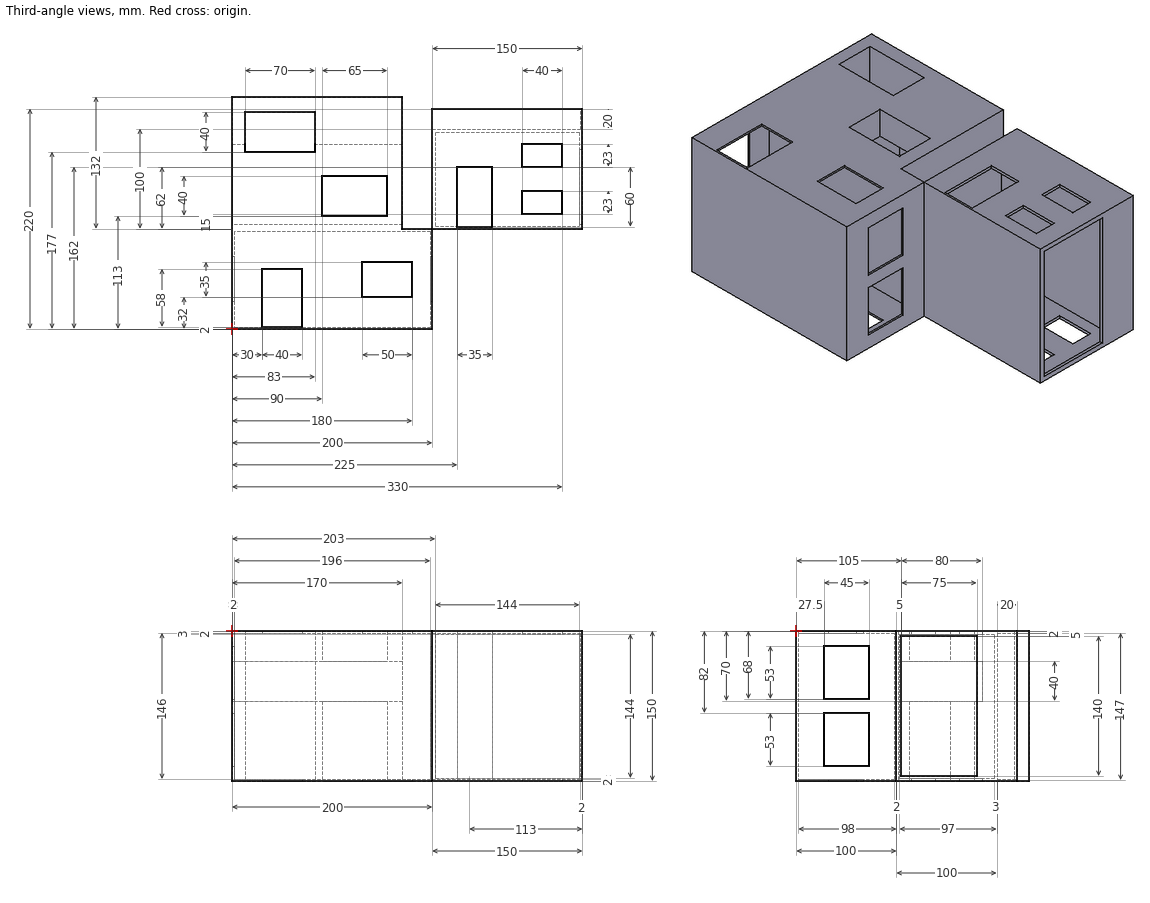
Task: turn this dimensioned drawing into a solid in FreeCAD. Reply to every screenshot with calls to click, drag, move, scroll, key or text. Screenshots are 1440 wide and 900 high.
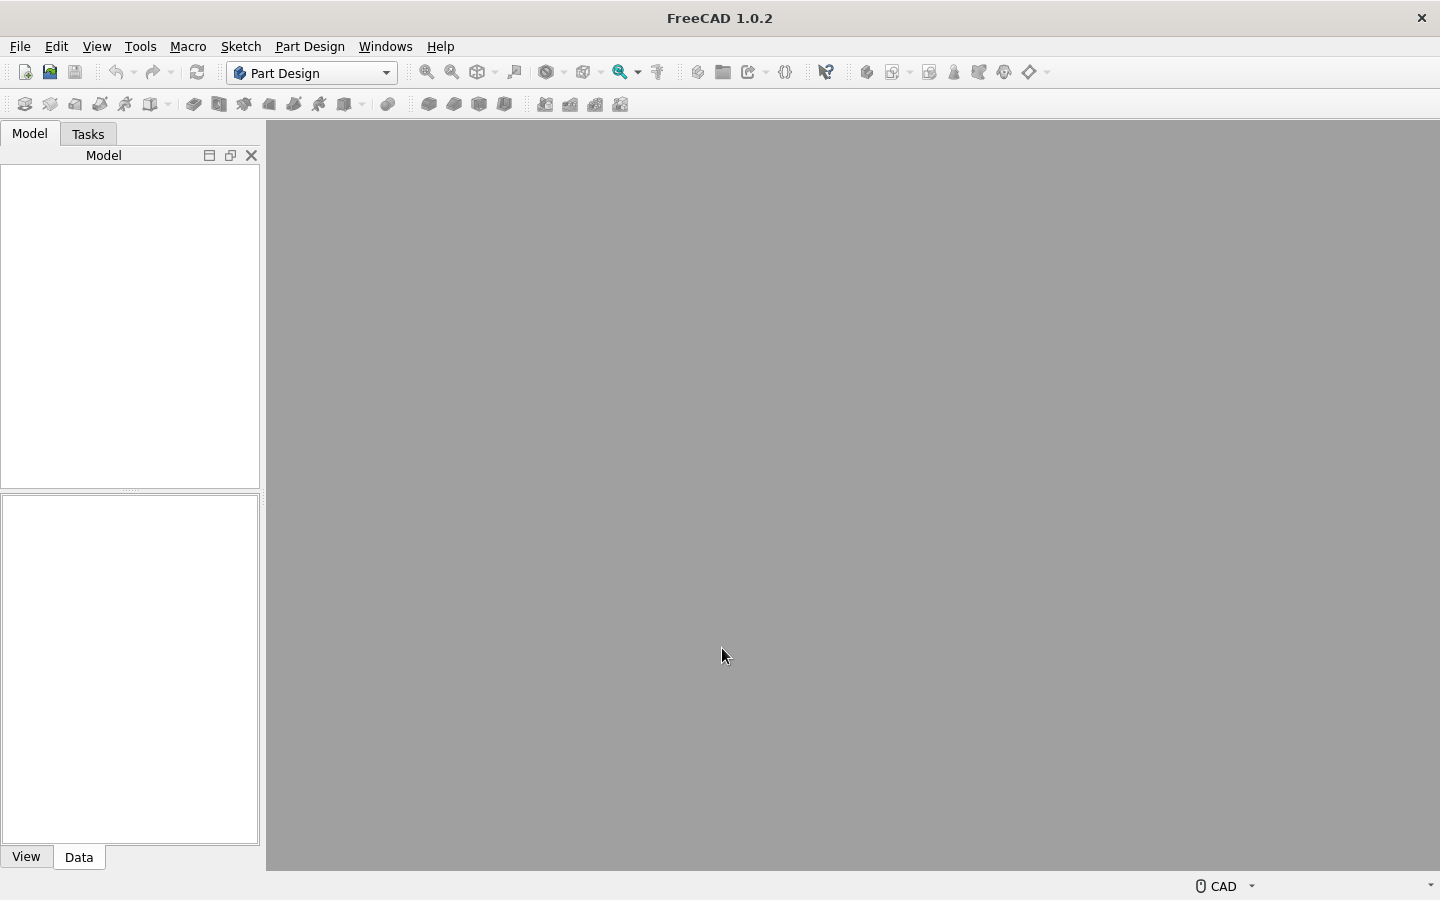
click(25, 72)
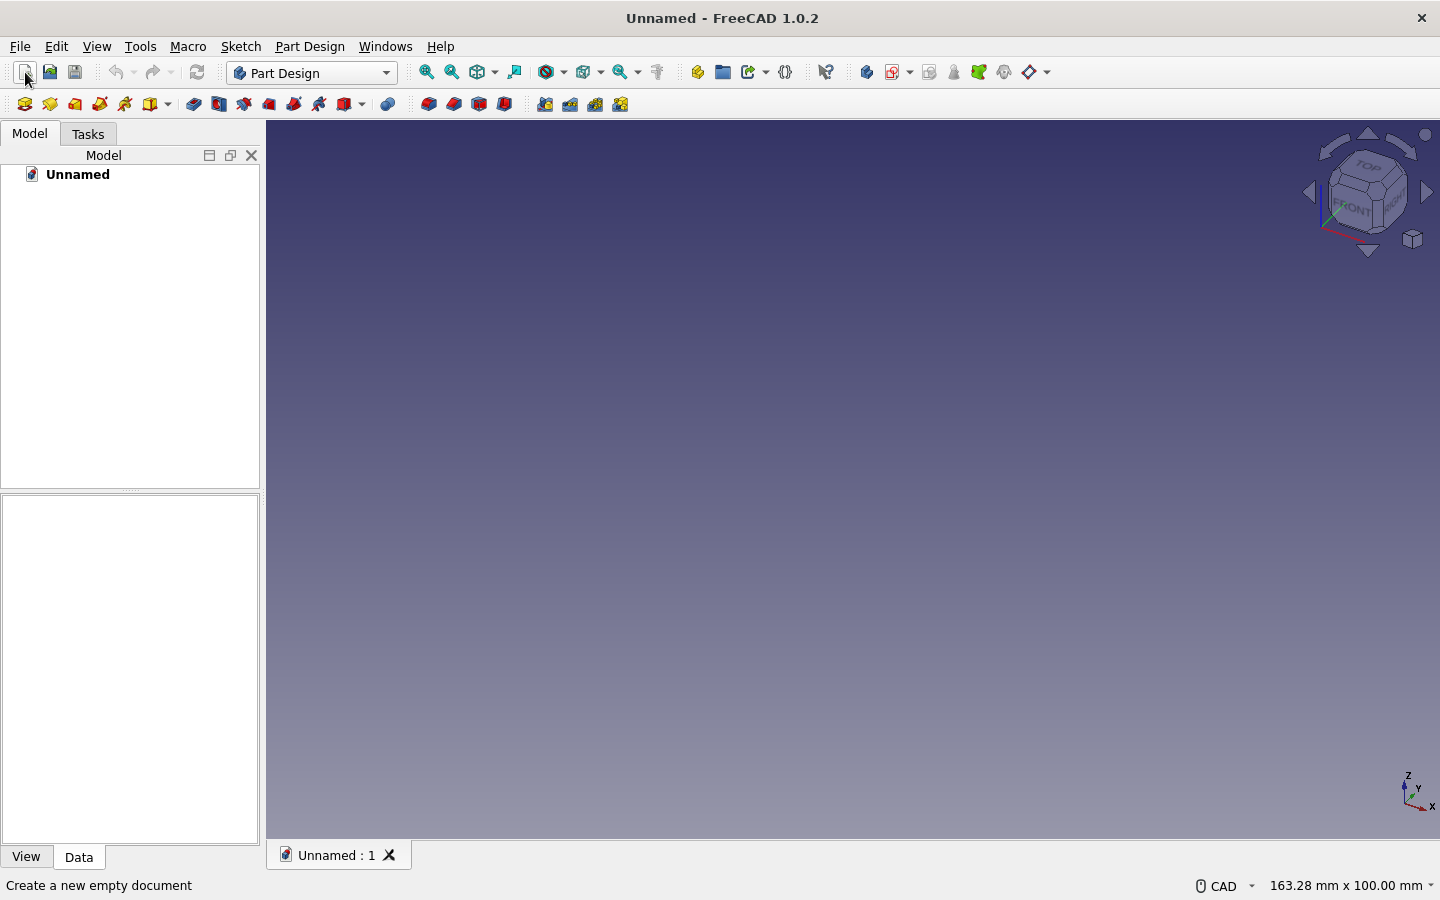
click(892, 72)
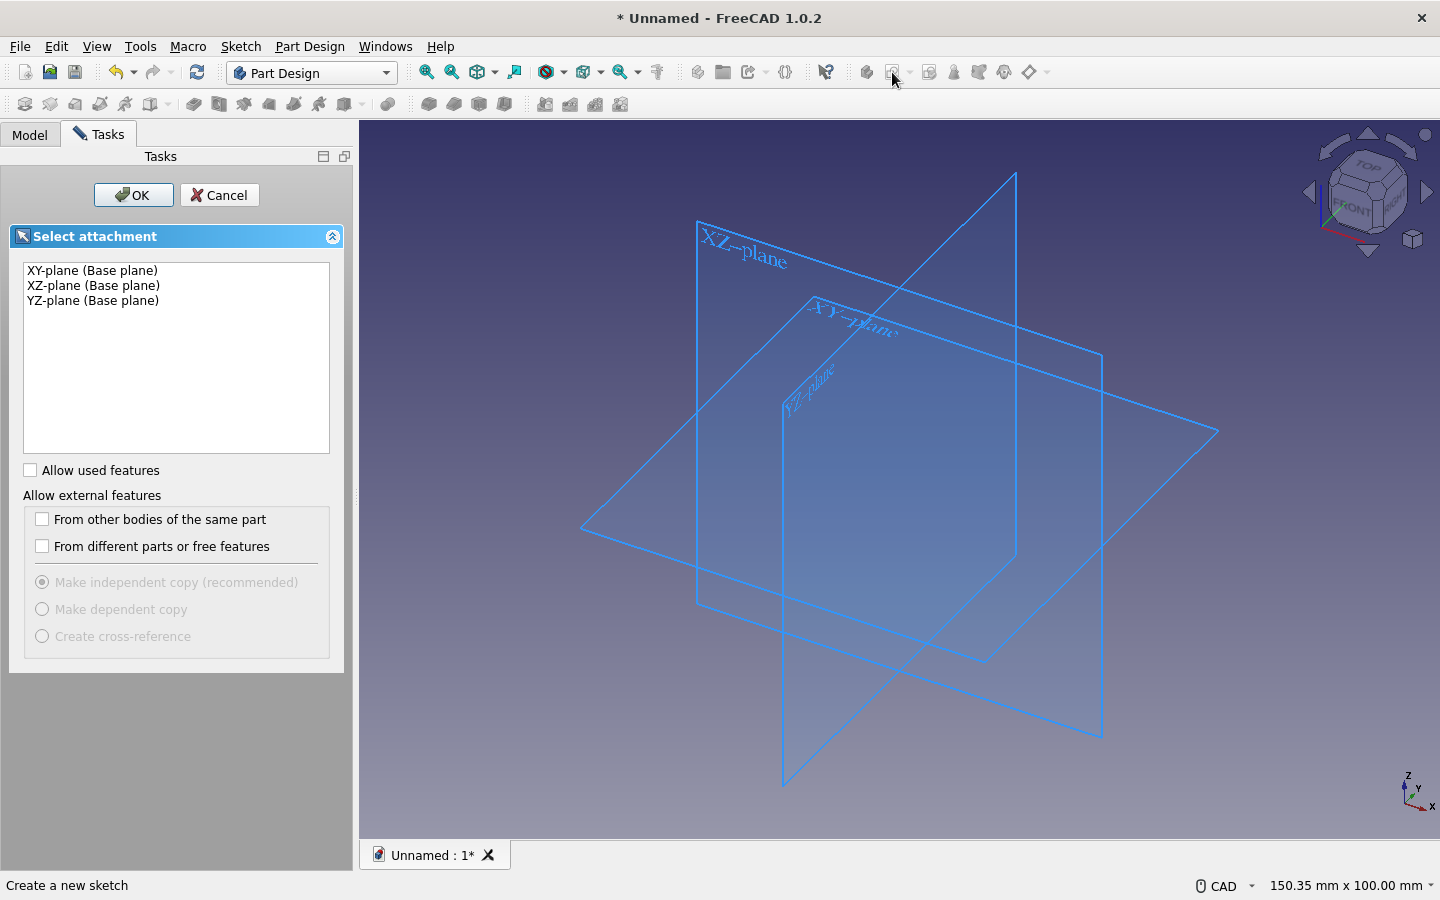
click(84, 286)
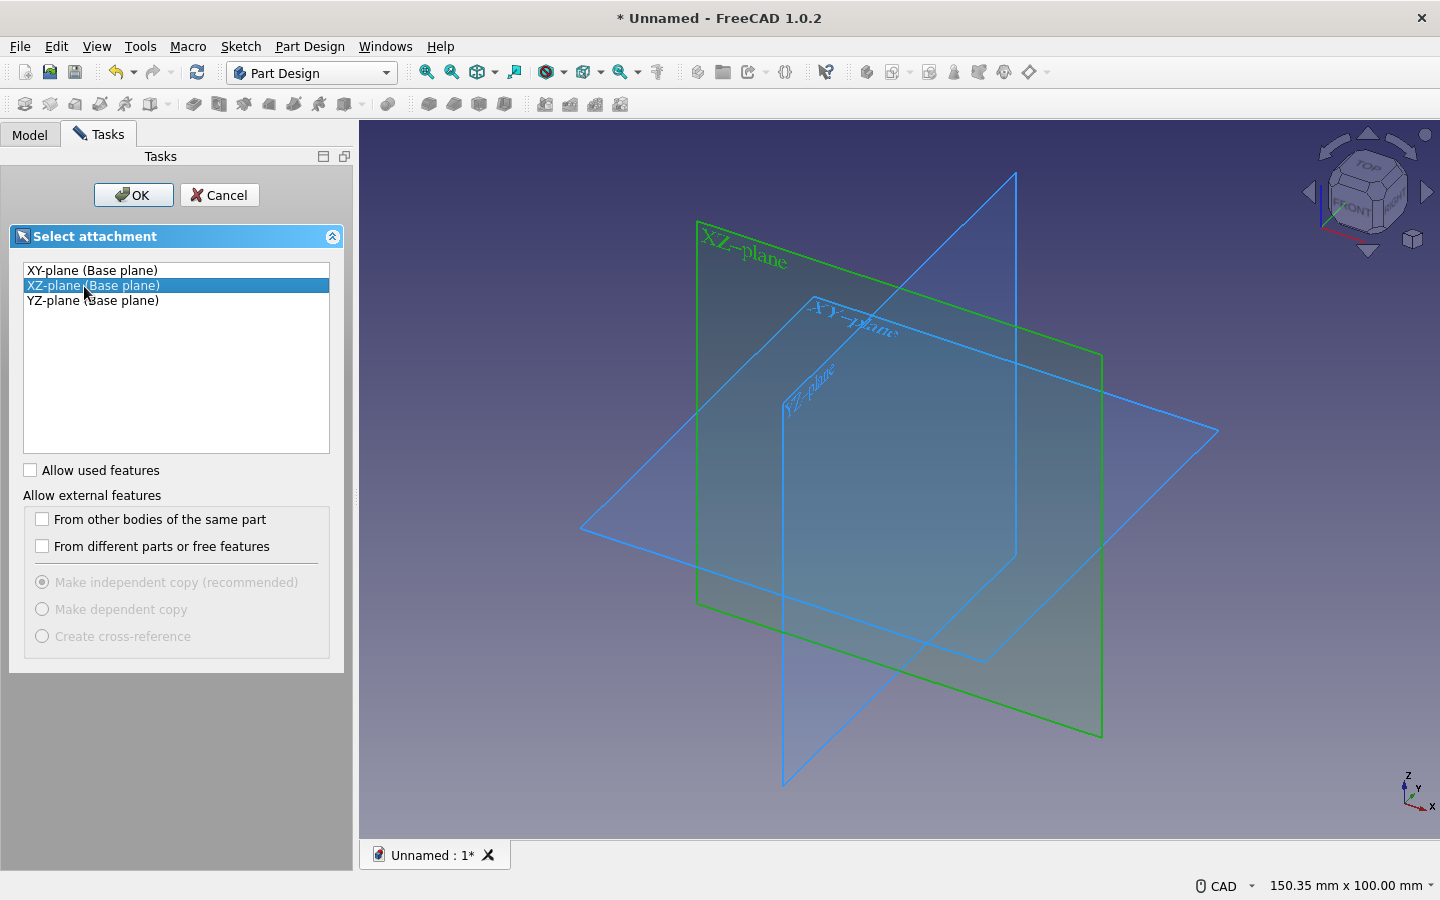
click(134, 195)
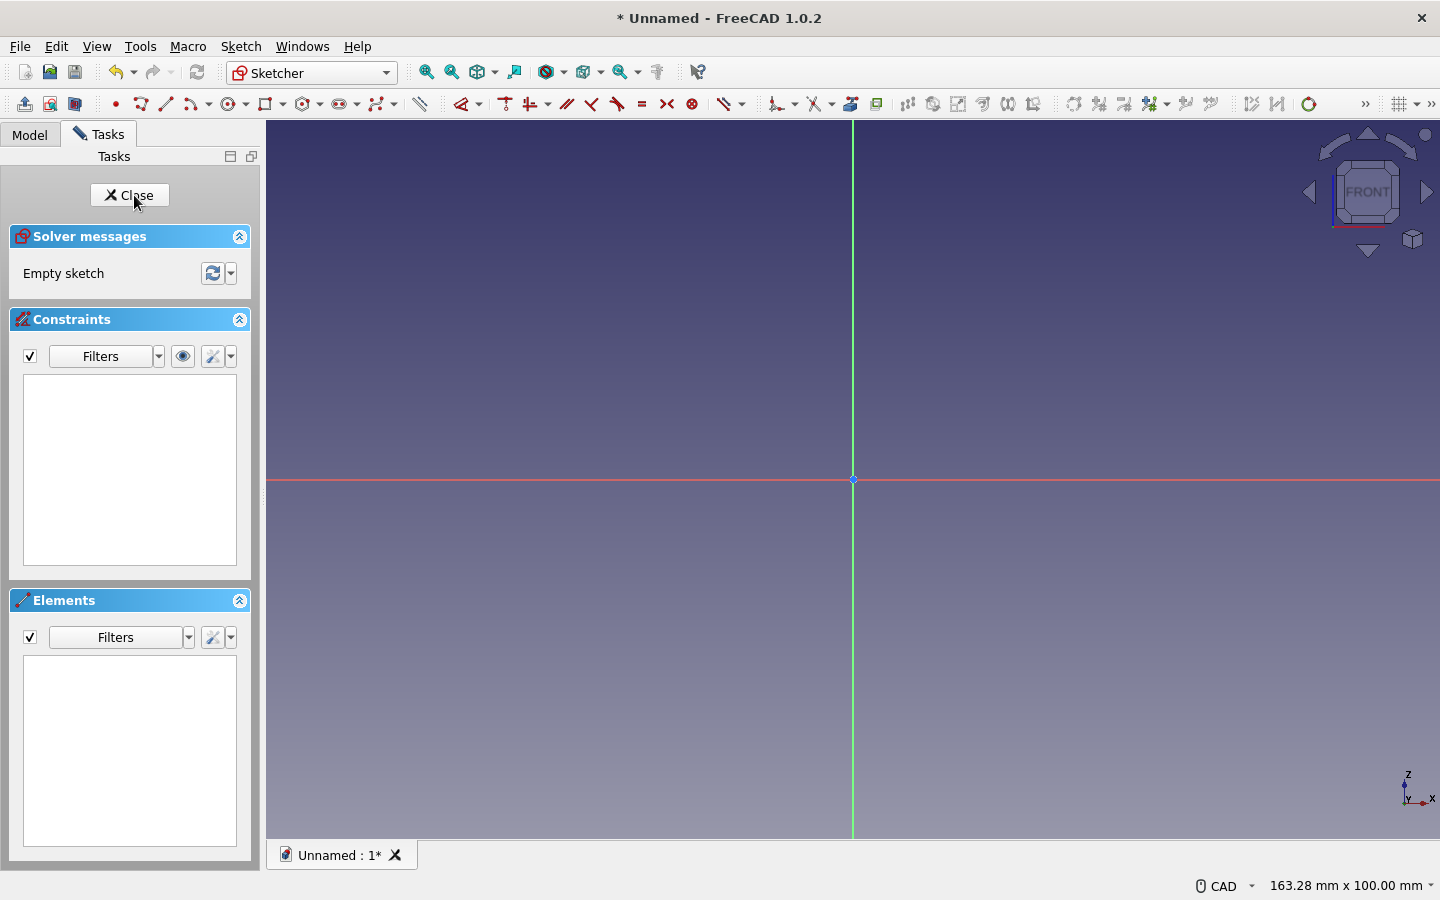
scroll(294, 148, down, 4)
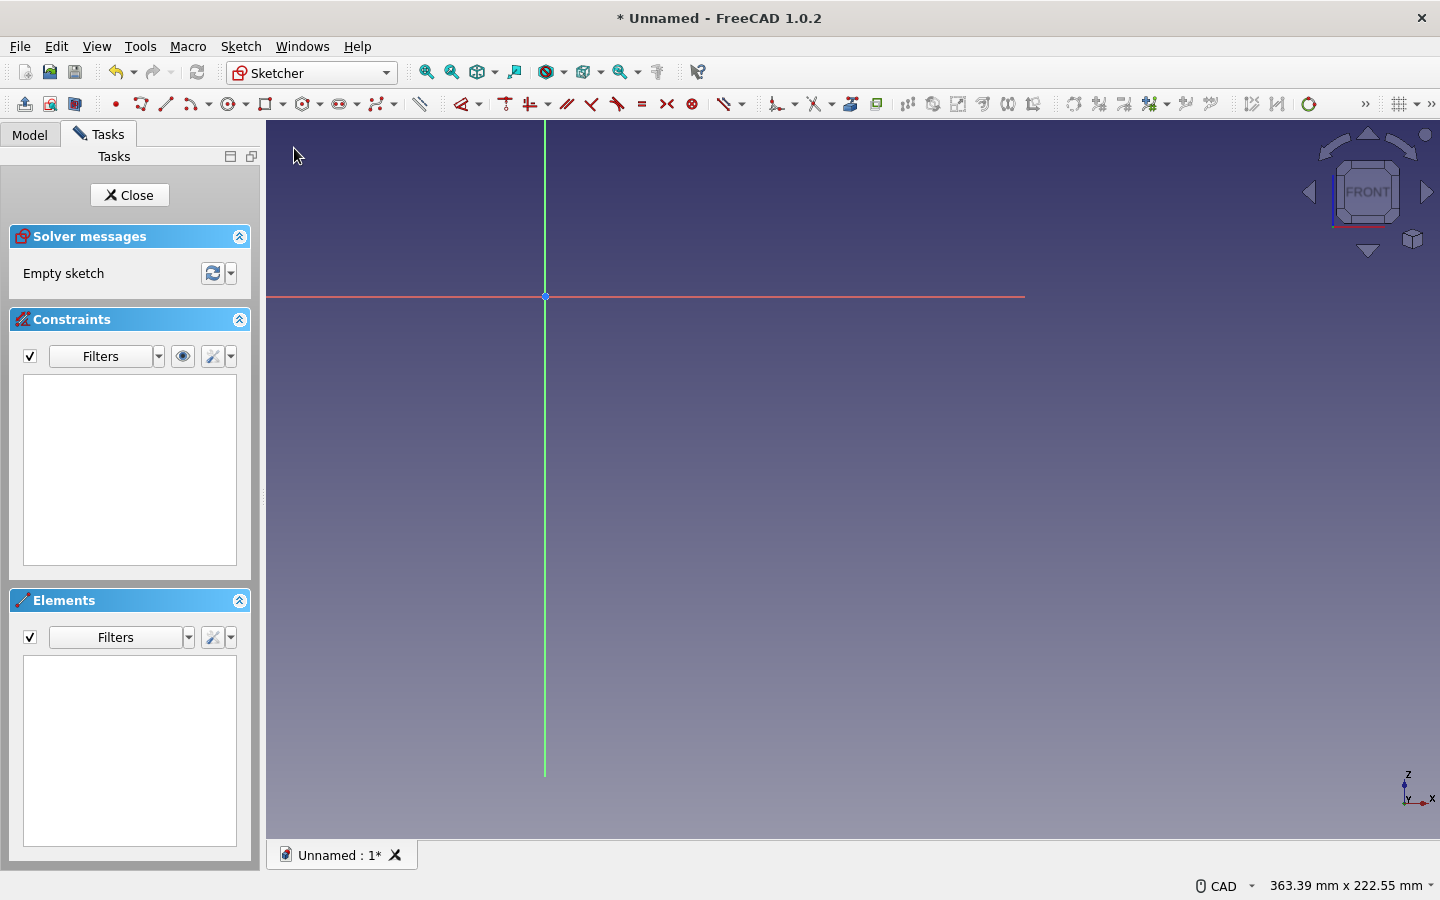
click(264, 104)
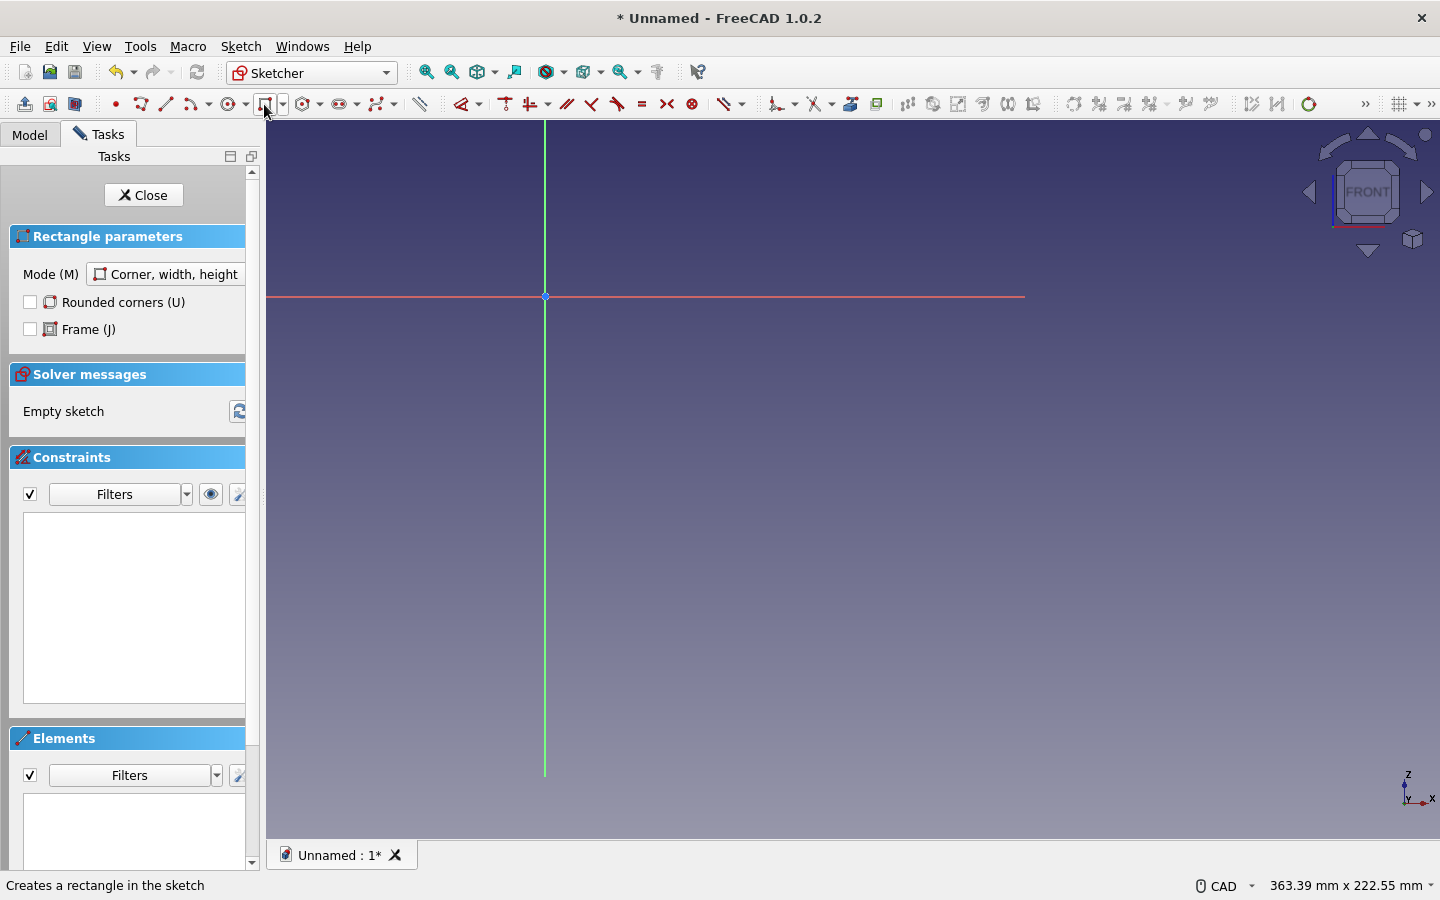
click(545, 297)
move(1191, 782)